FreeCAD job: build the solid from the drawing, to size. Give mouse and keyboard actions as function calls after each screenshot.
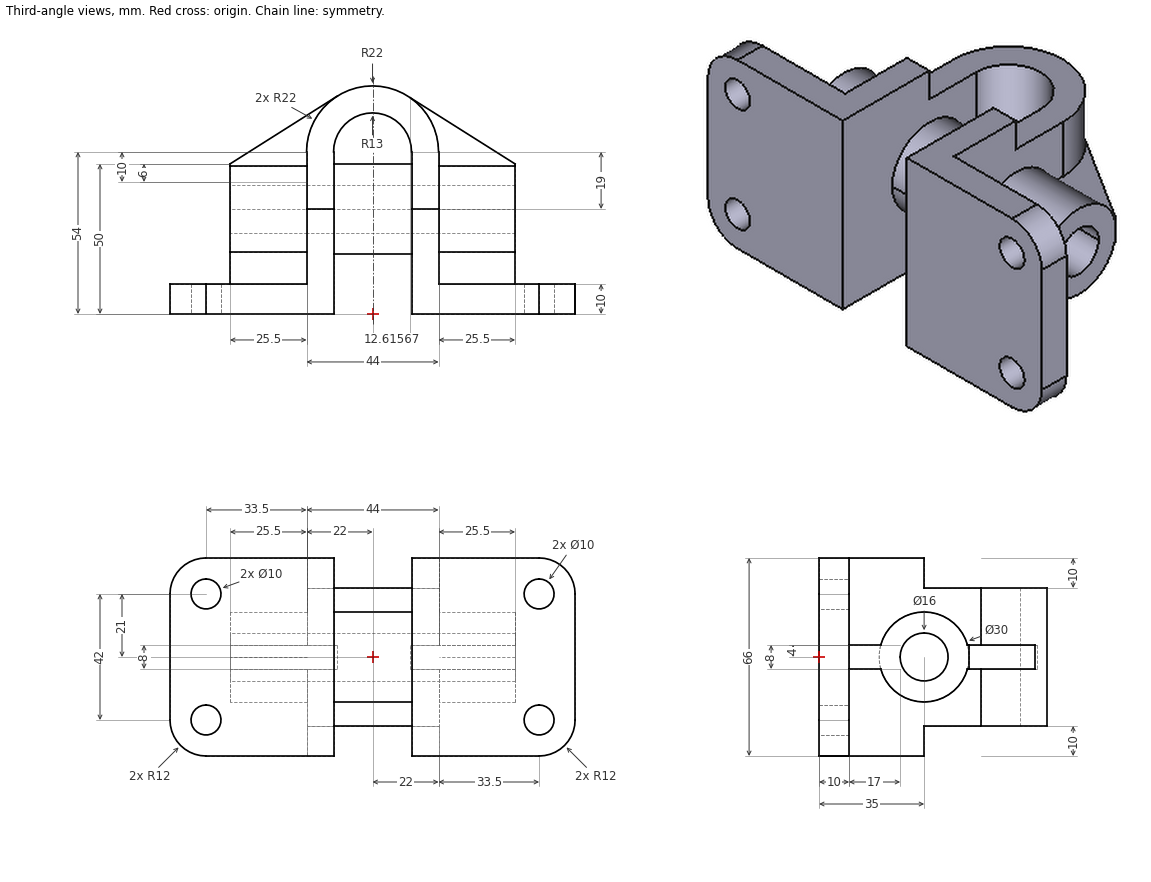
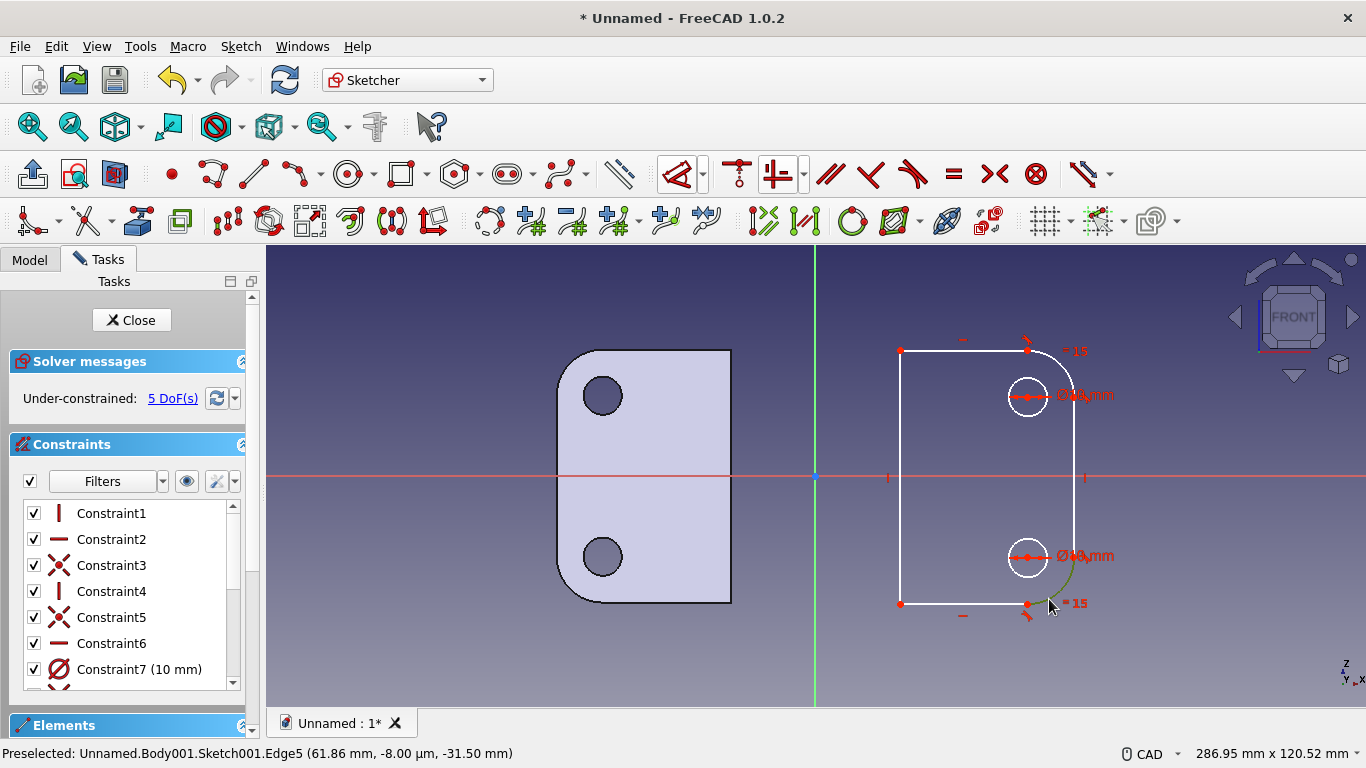
key(k)
key(r)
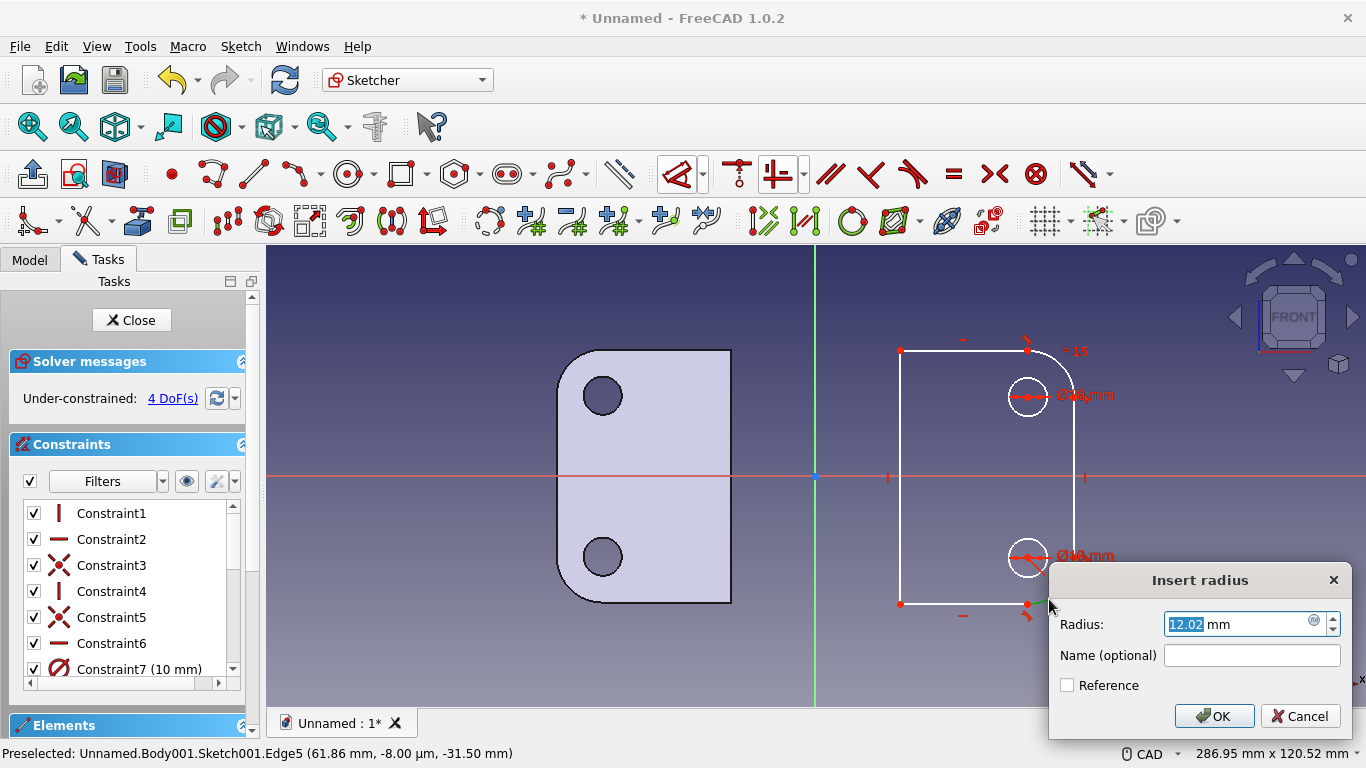
text(12)
key(Return)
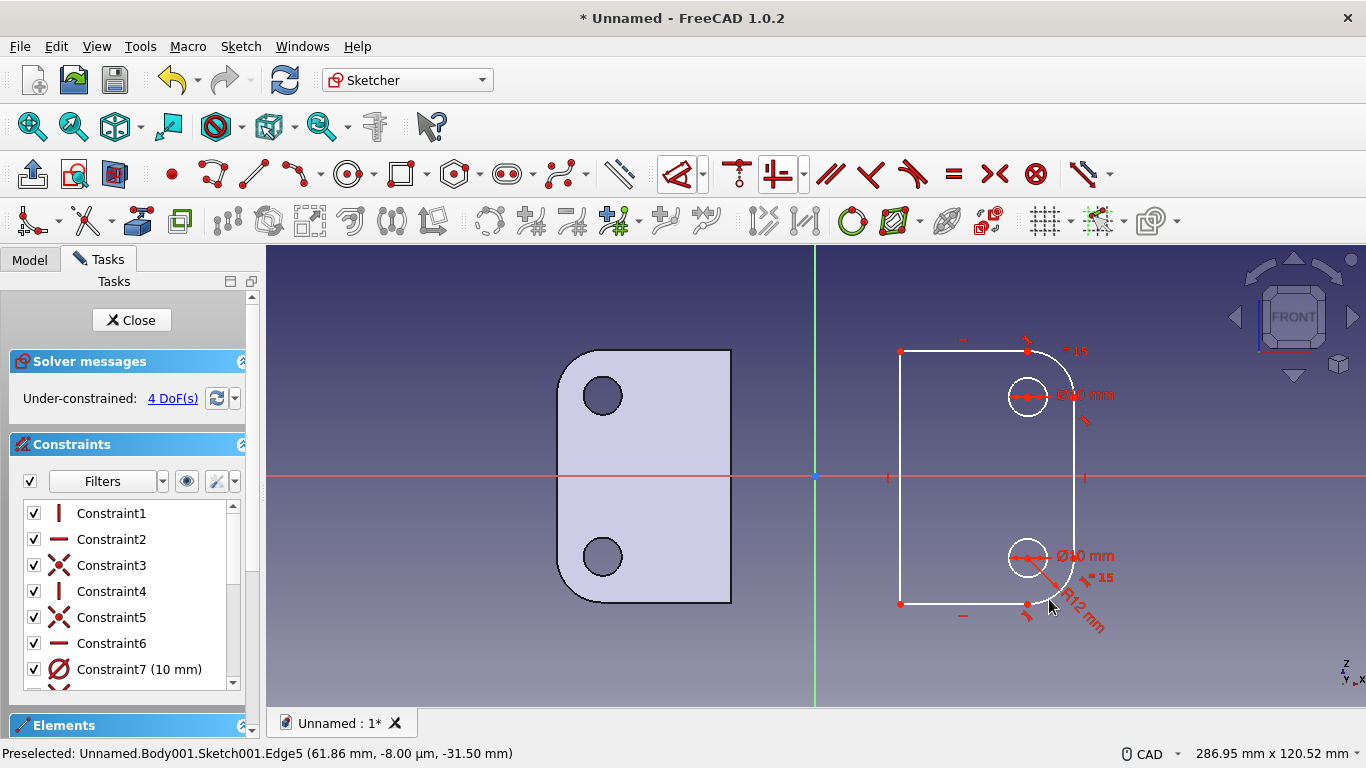
click(1074, 445)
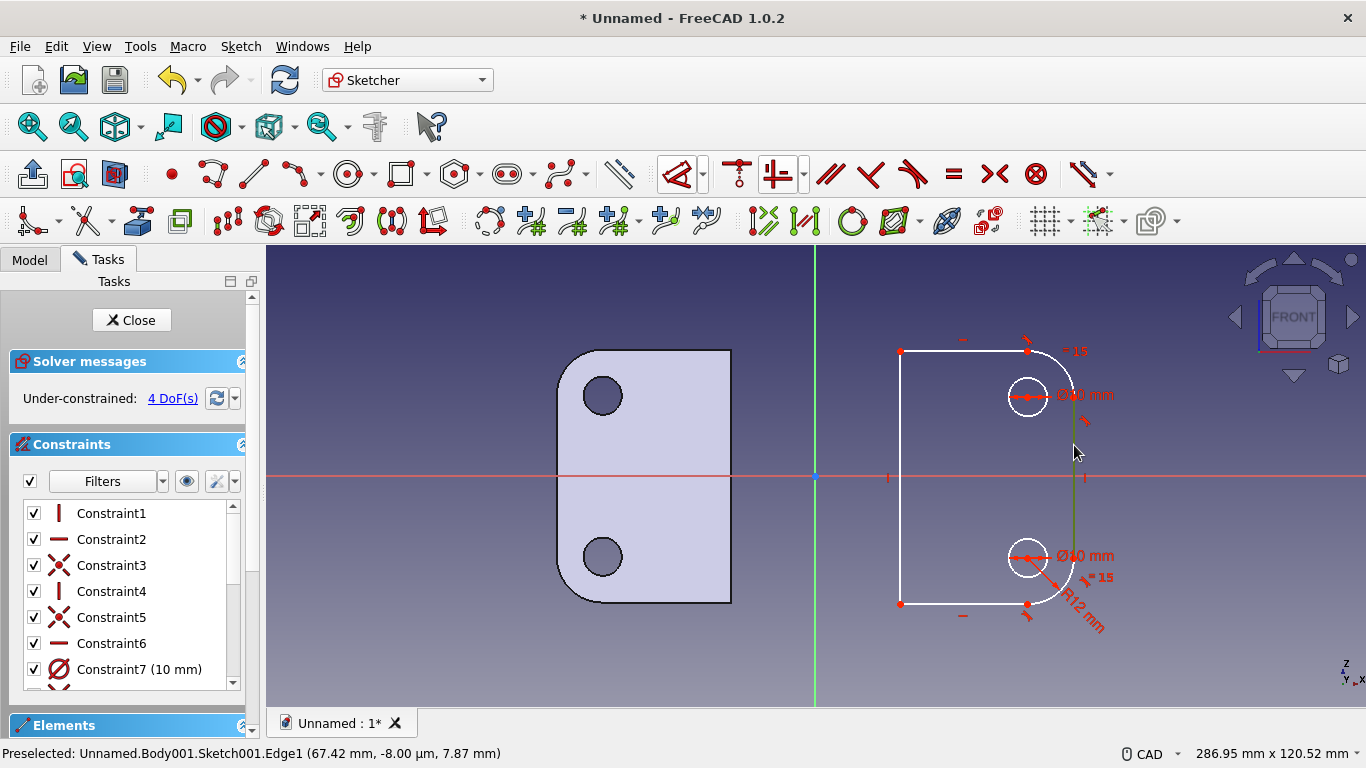
key(i)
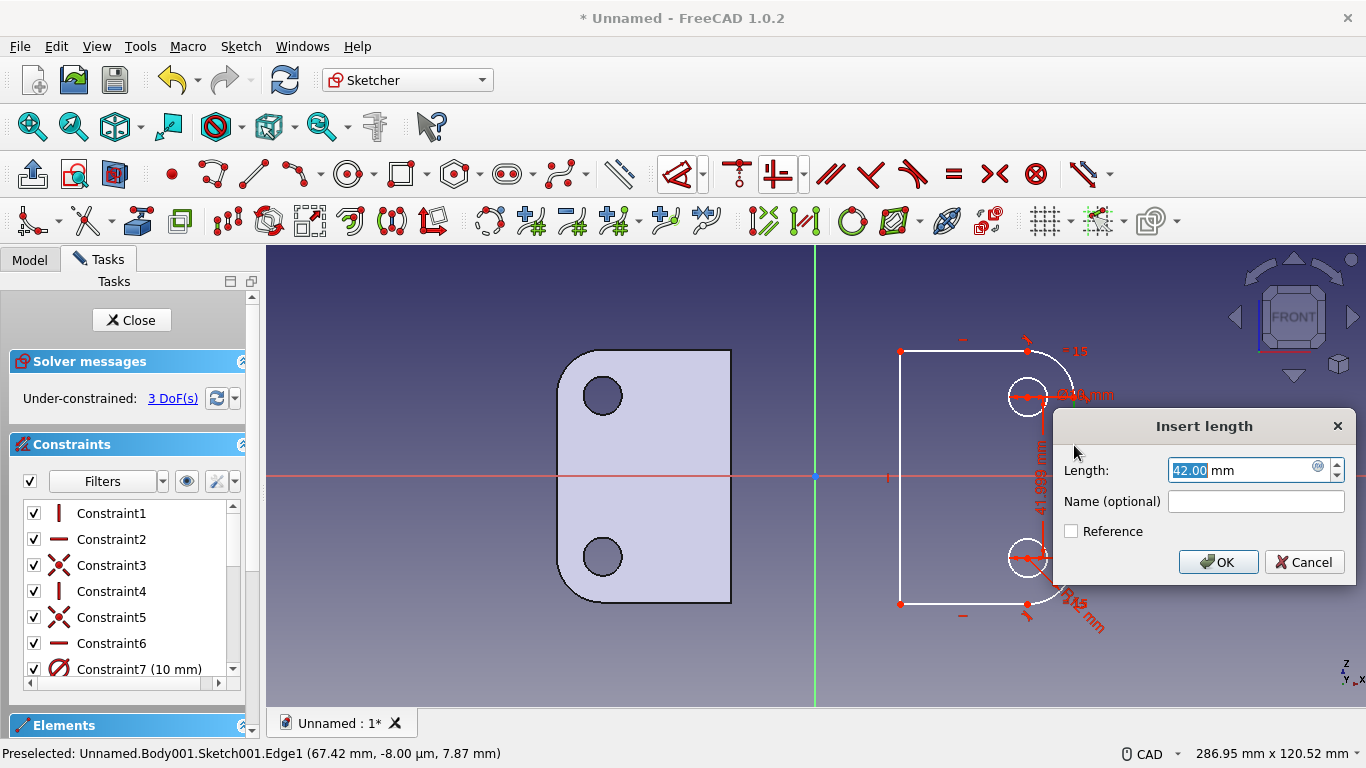
text(42)
key(Return)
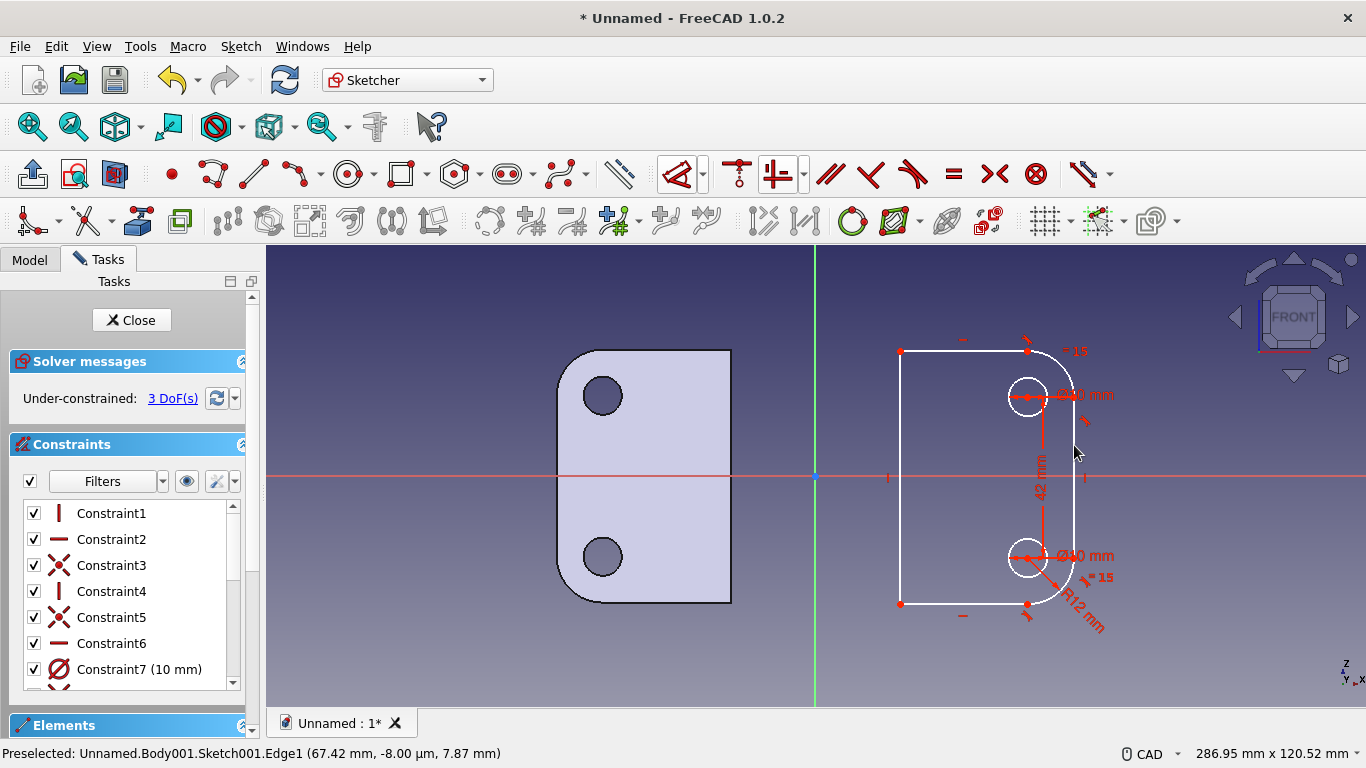
click(1028, 397)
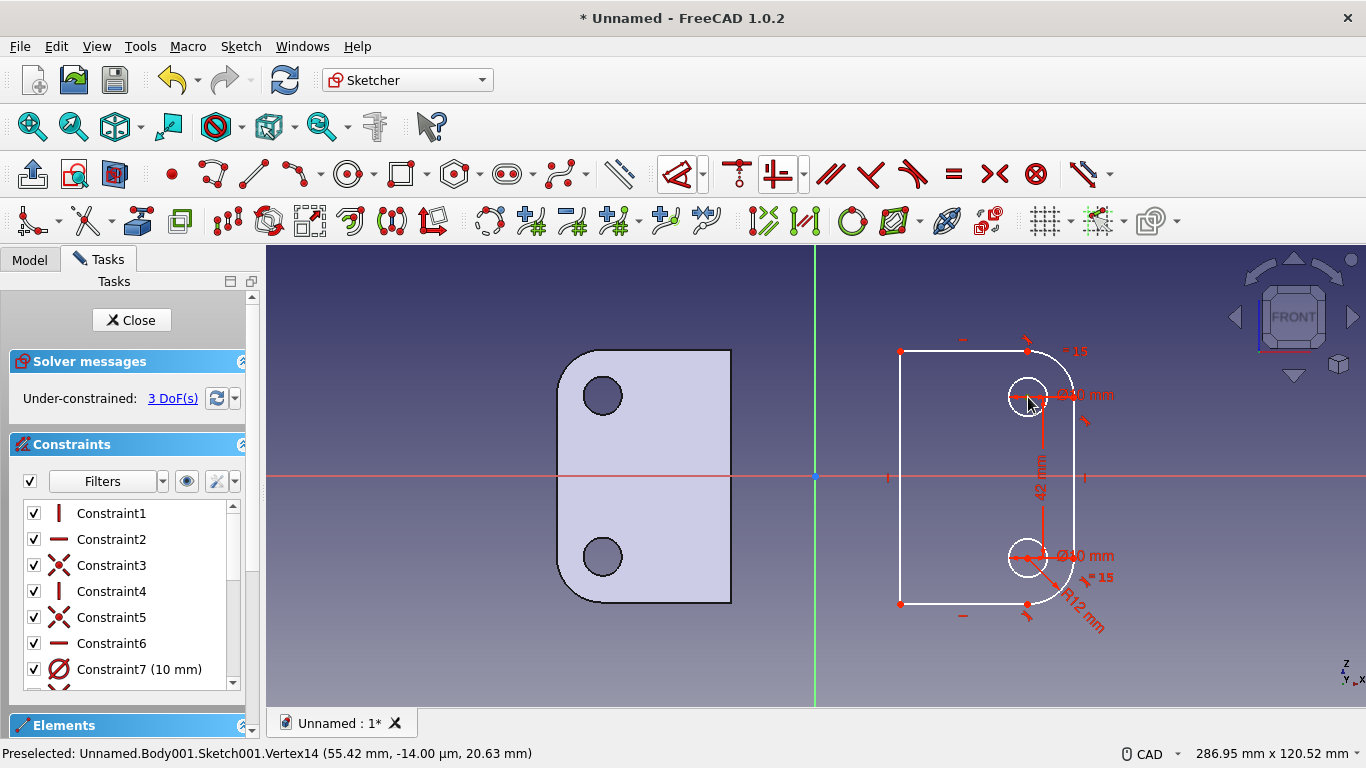
click(702, 174)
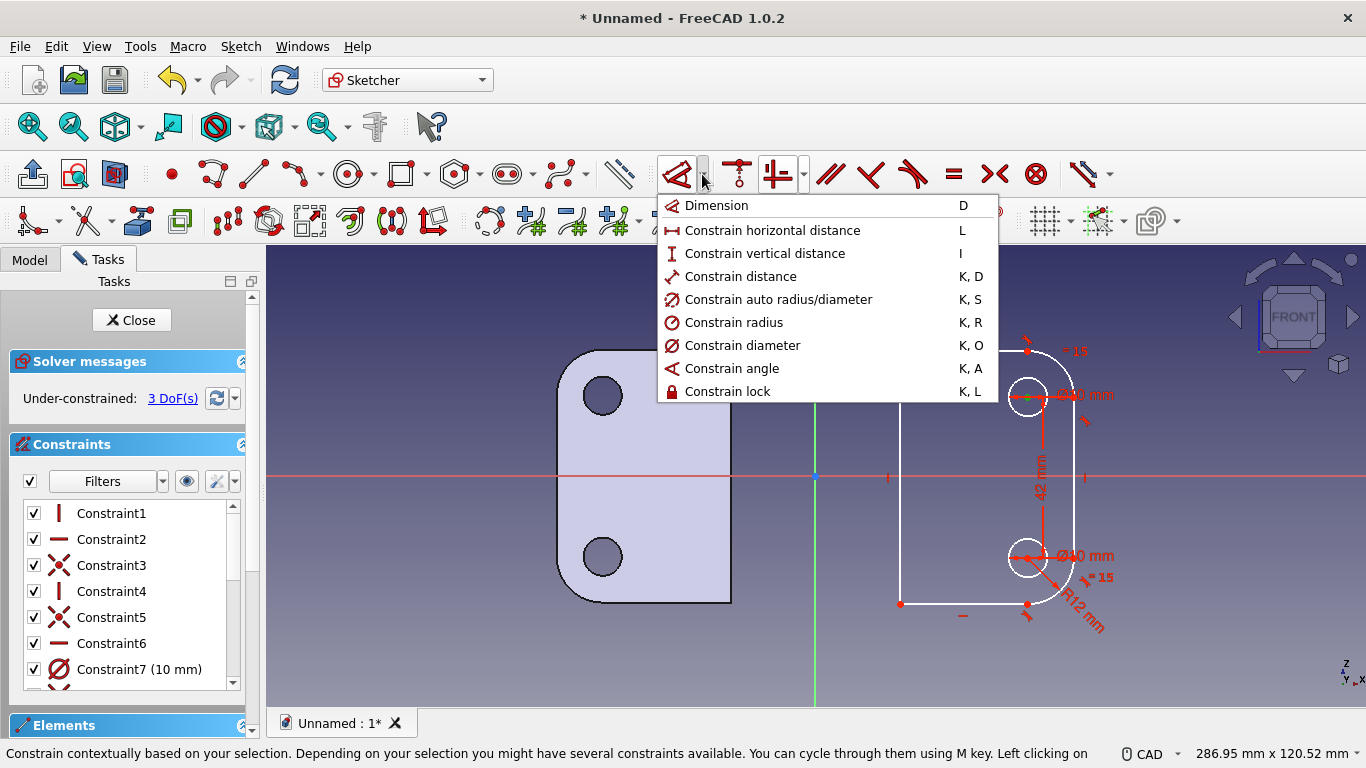
click(828, 254)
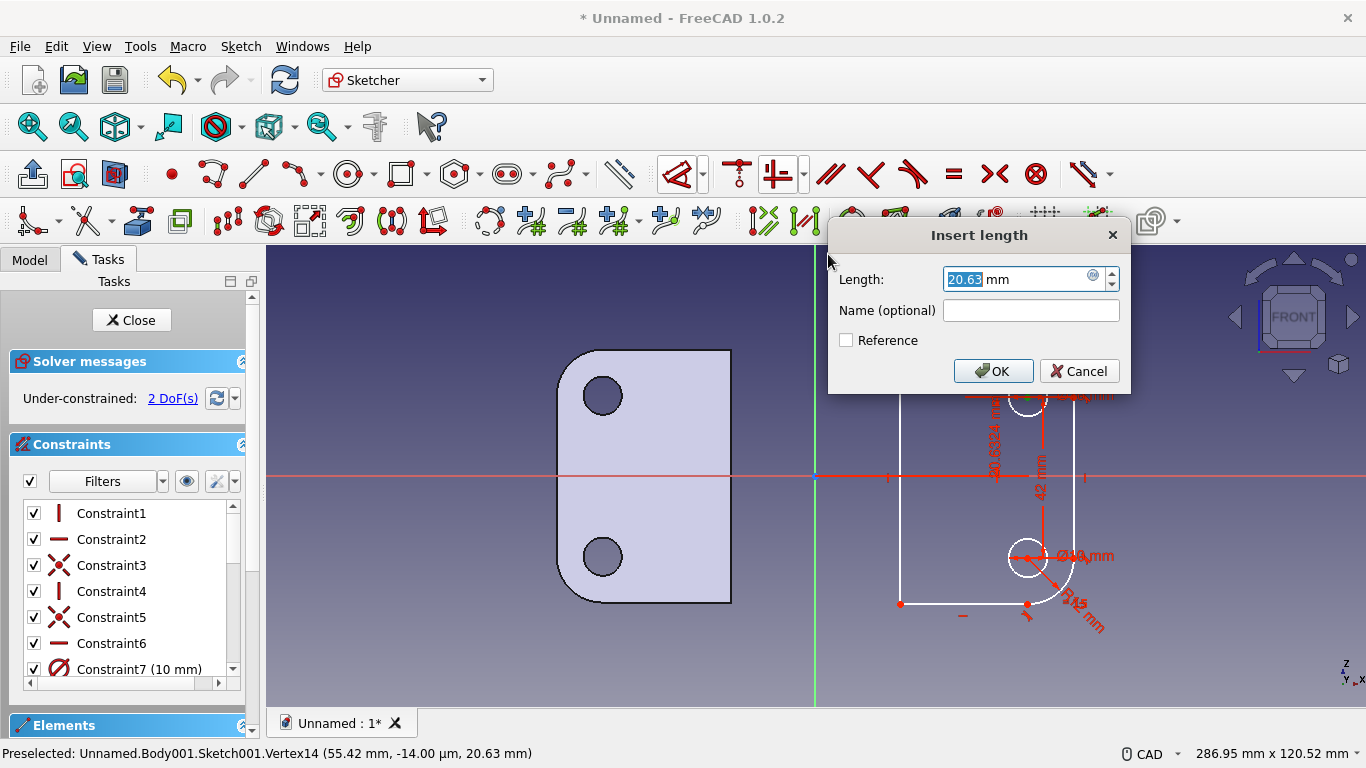
text(21)
key(Return)